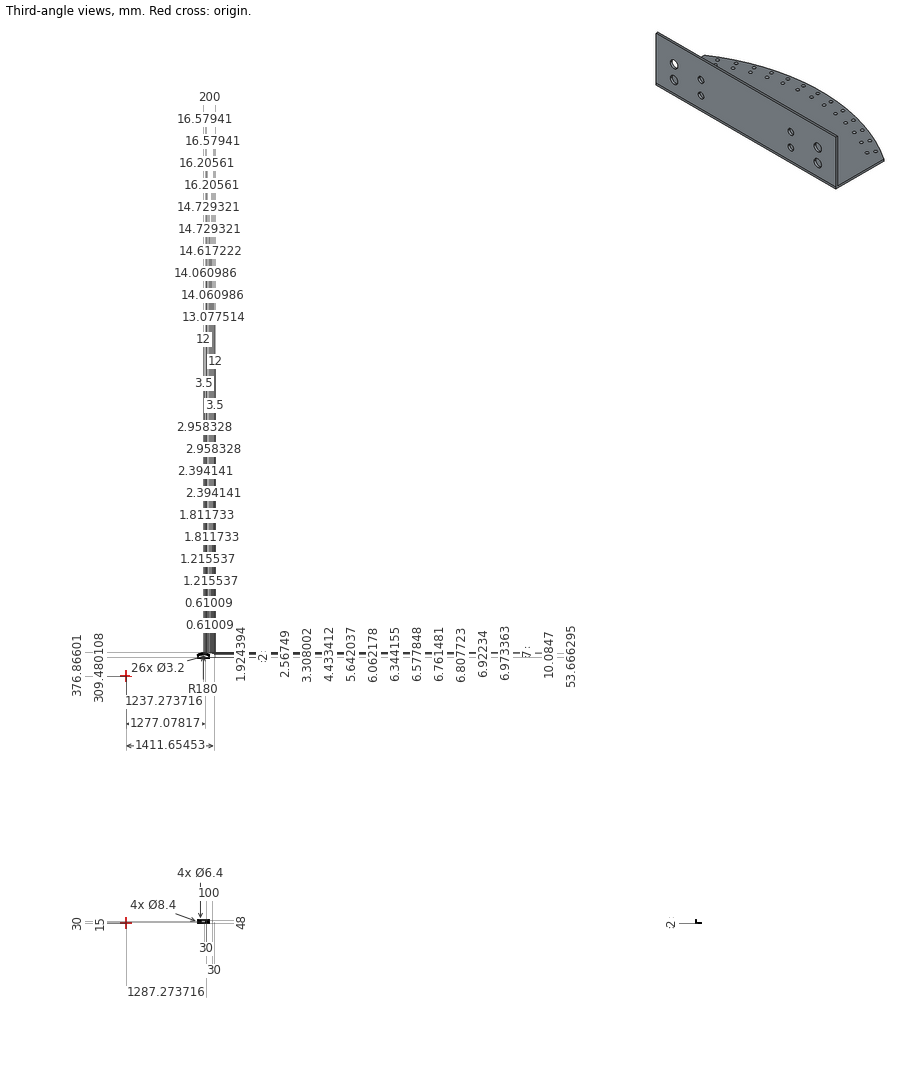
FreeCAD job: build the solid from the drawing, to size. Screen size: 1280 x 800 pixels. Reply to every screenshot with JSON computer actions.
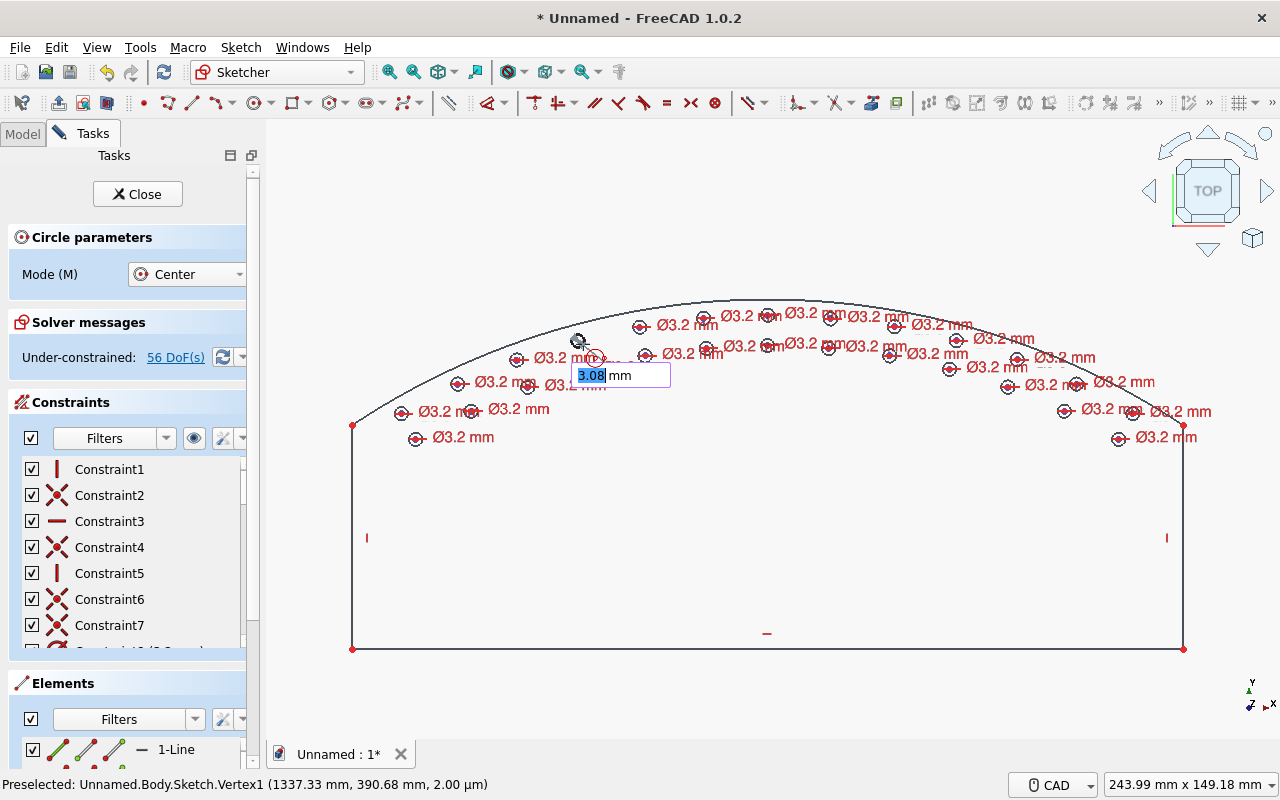
{"action": "type", "text": "3.2"}
{"action": "key", "text": "Return"}
{"action": "key", "text": "Escape"}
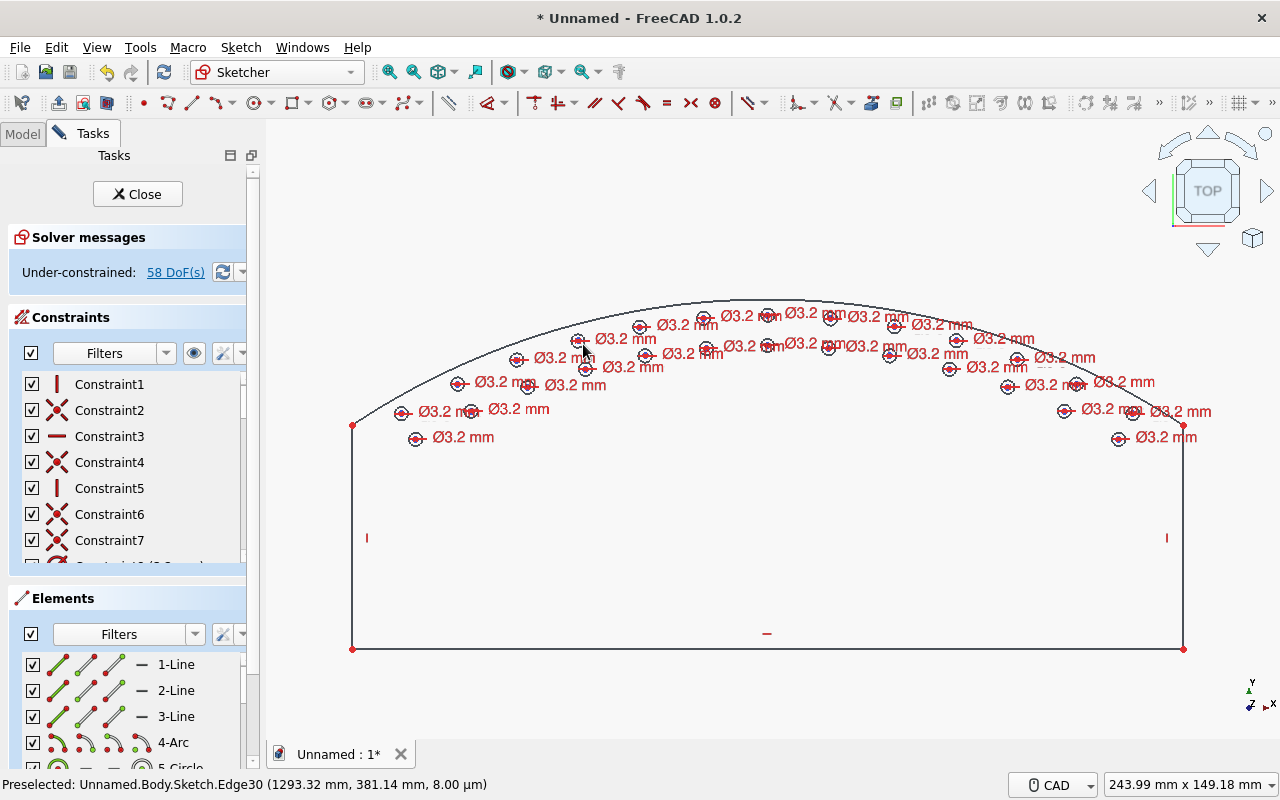
{"action": "left_click", "coordinate": [768, 345]}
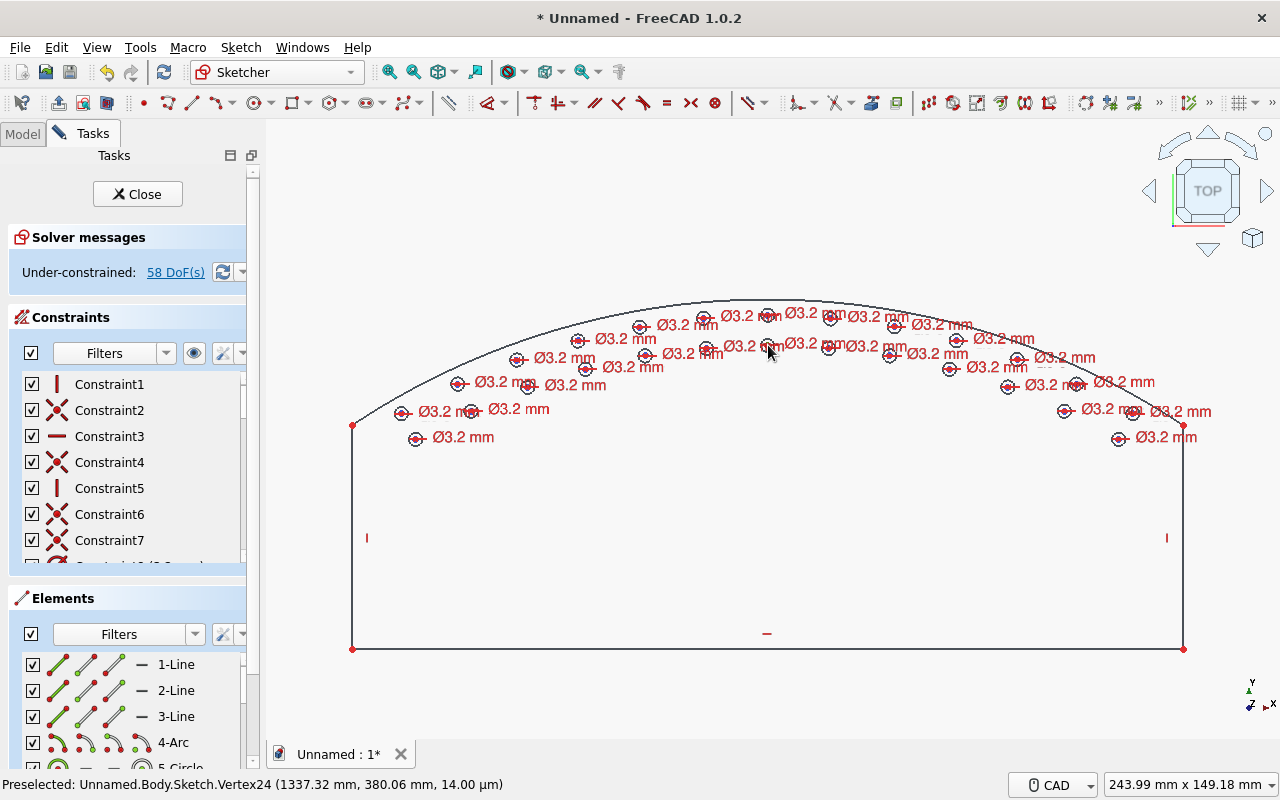
{"action": "left_click", "coordinate": [768, 315]}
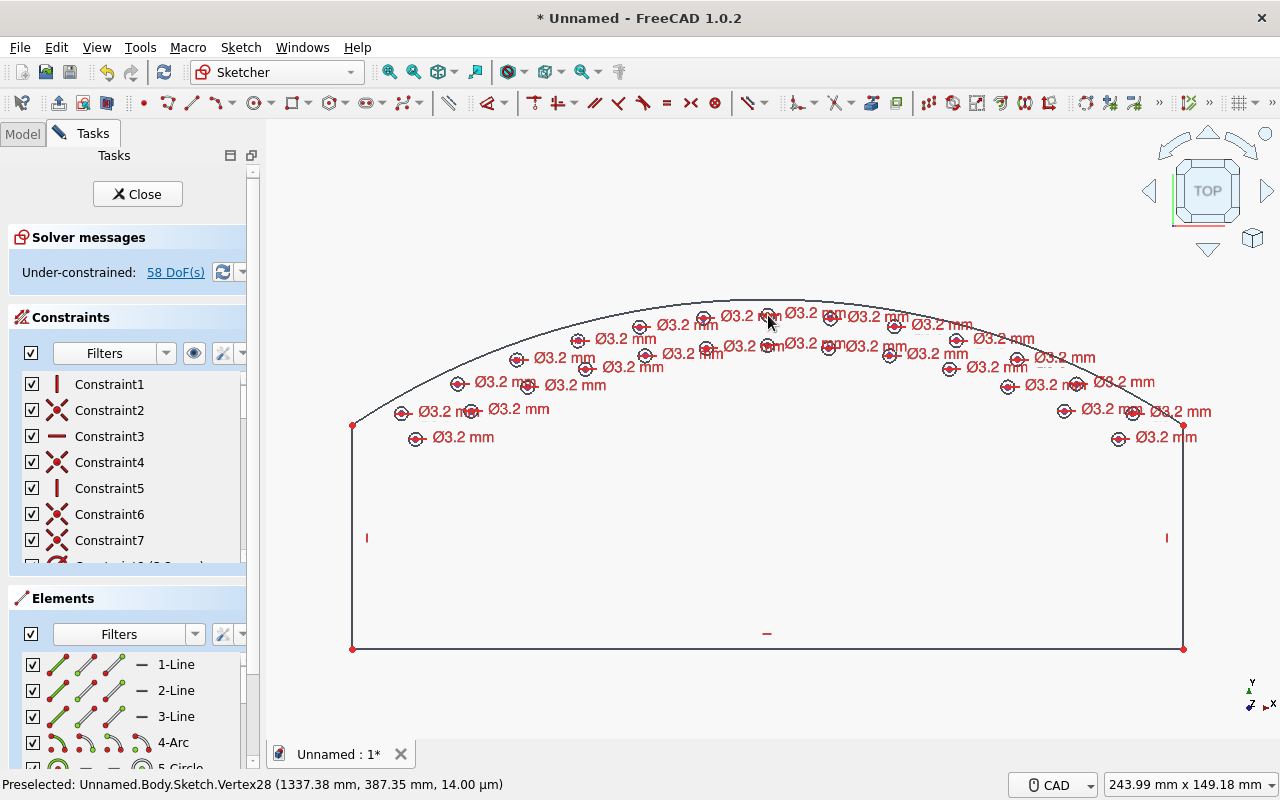
{"action": "key", "text": "v"}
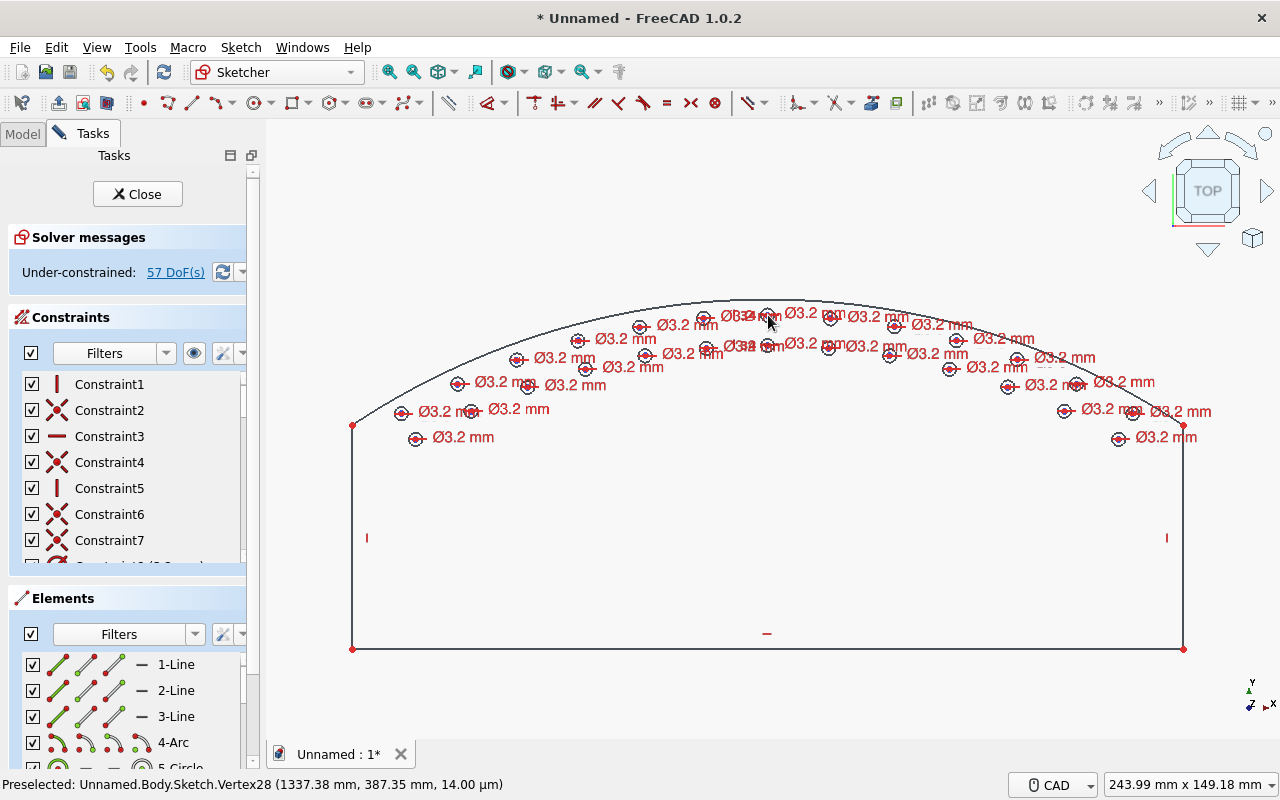
{"action": "left_click", "coordinate": [829, 348]}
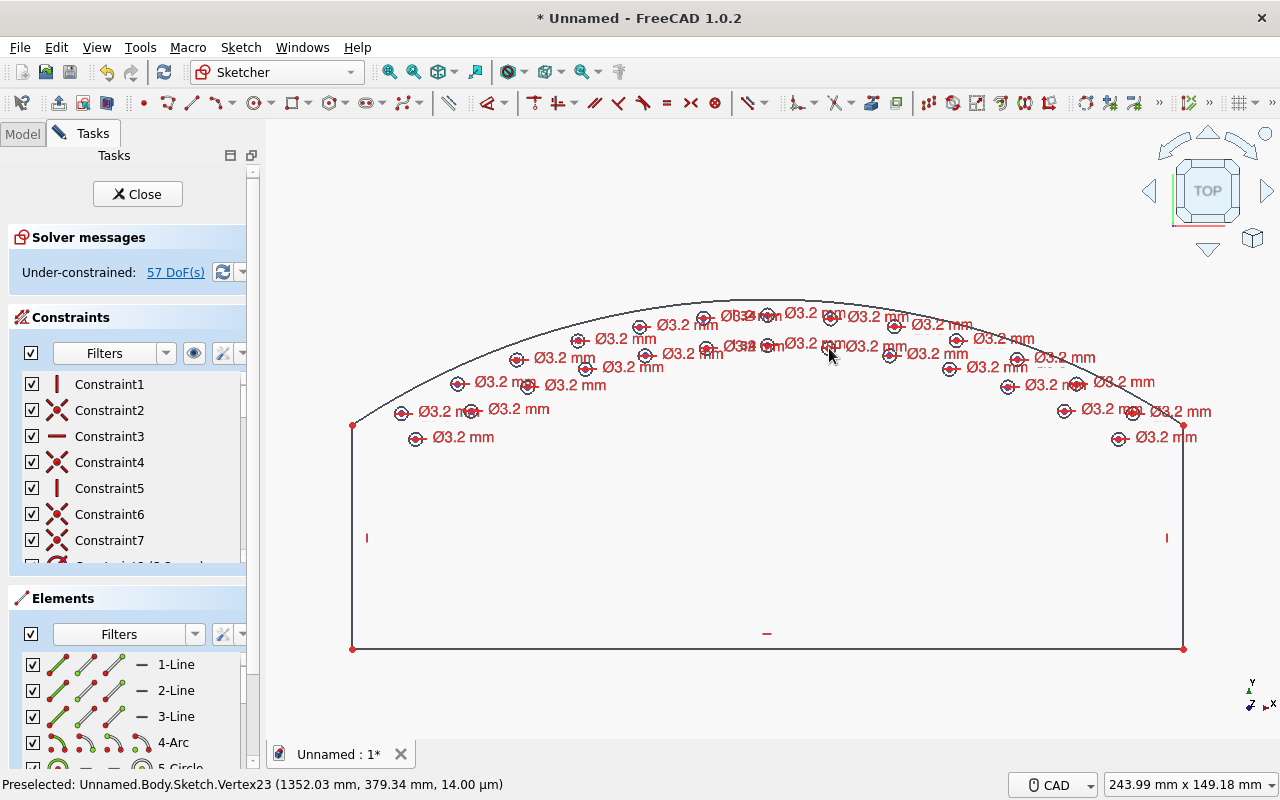
{"action": "left_click", "coordinate": [706, 348]}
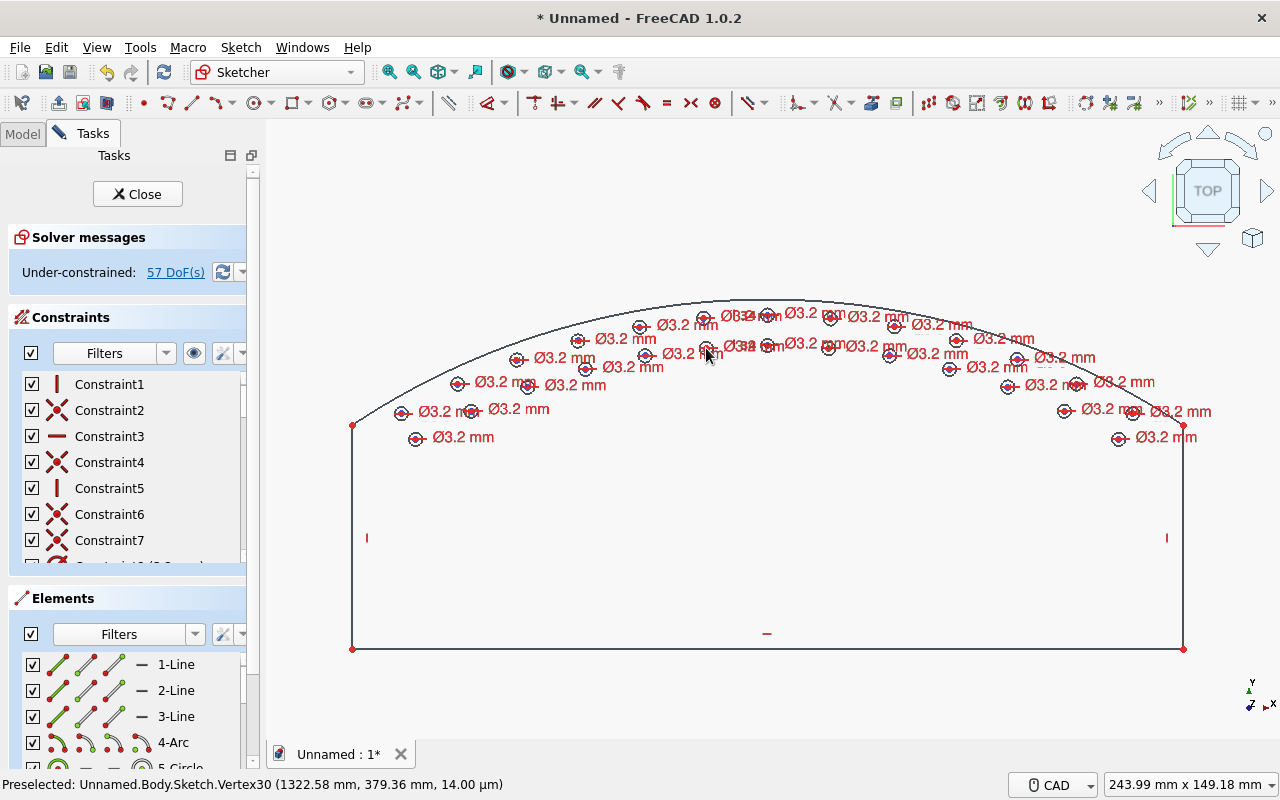
{"action": "left_click", "coordinate": [576, 104]}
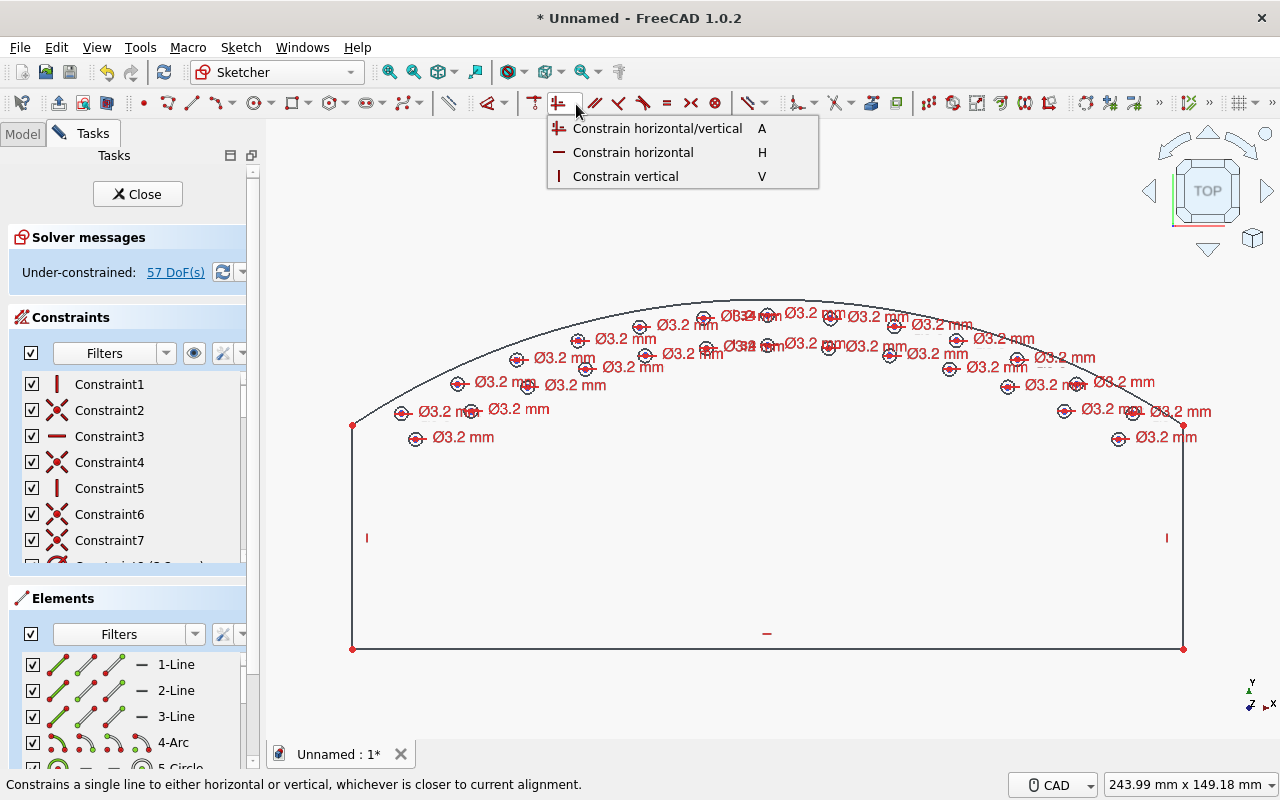
{"action": "left_click", "coordinate": [683, 152]}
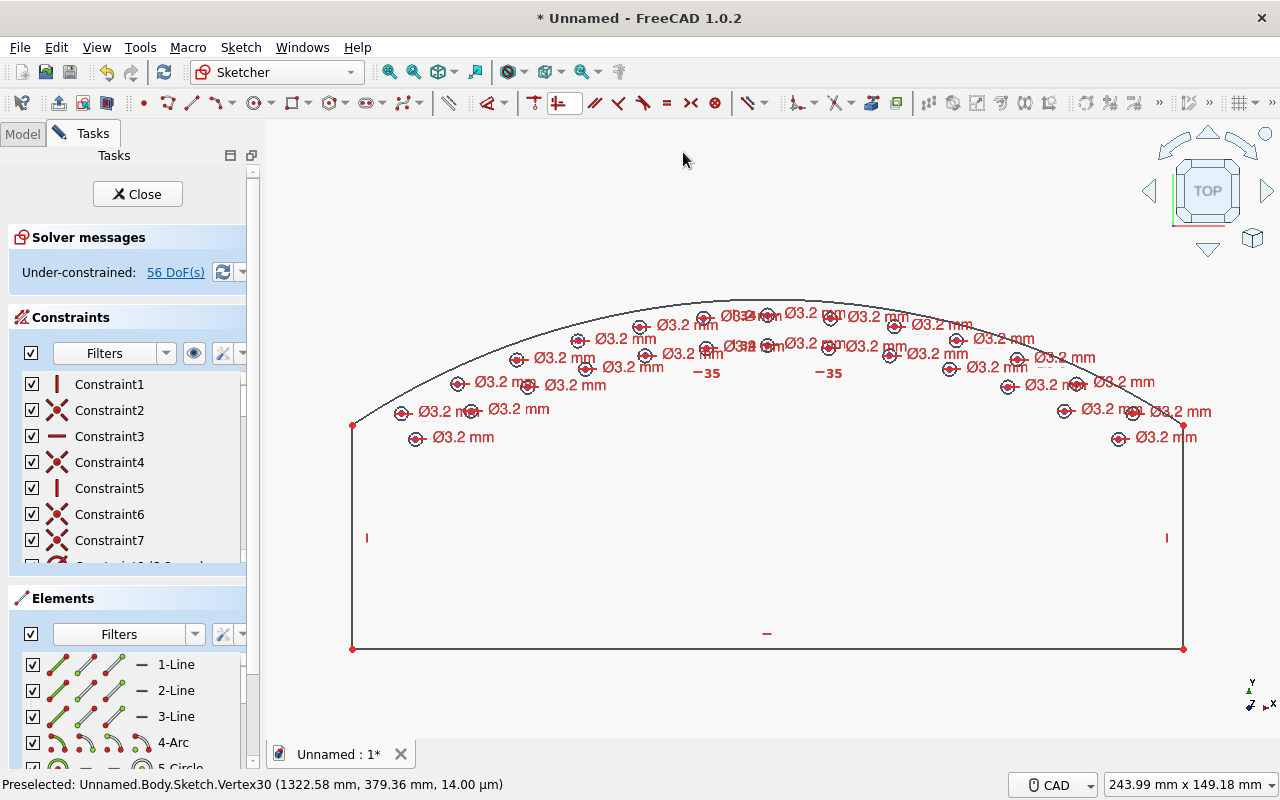
{"action": "left_click", "coordinate": [831, 319]}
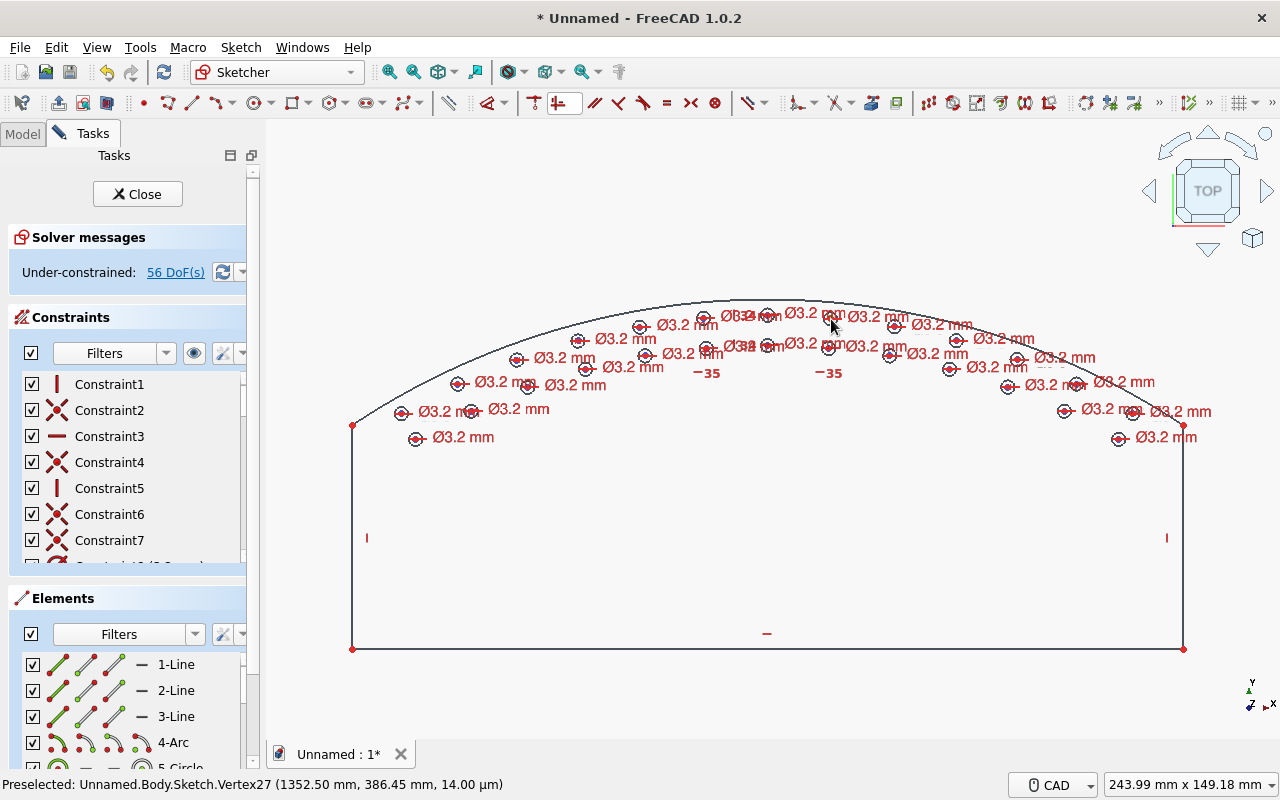
{"action": "left_click", "coordinate": [704, 318]}